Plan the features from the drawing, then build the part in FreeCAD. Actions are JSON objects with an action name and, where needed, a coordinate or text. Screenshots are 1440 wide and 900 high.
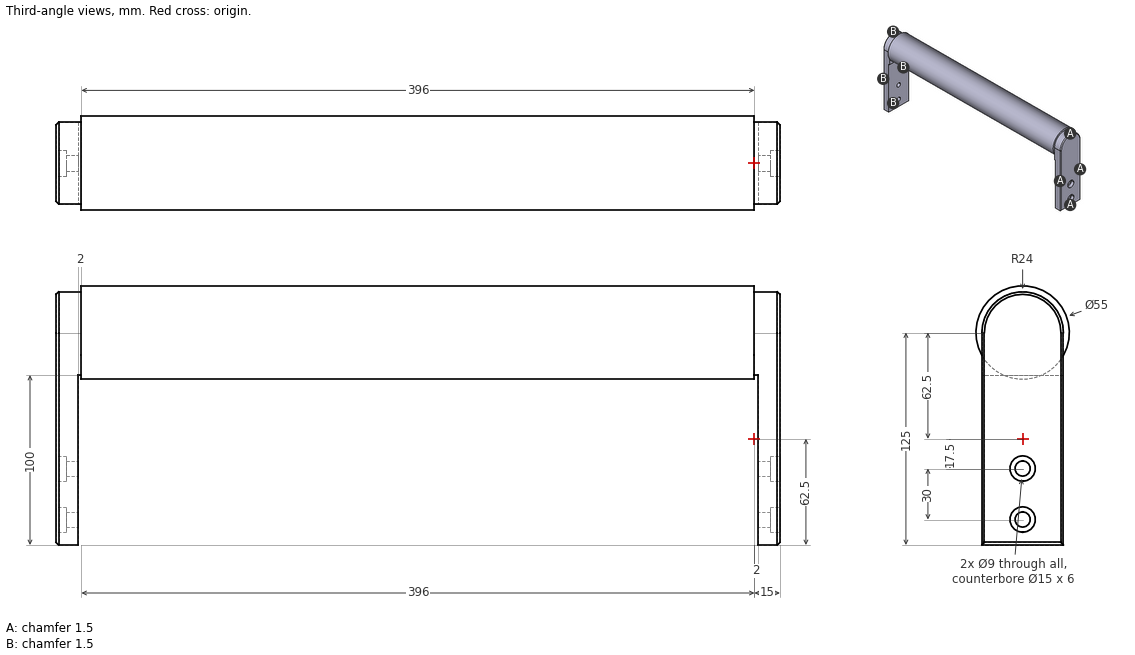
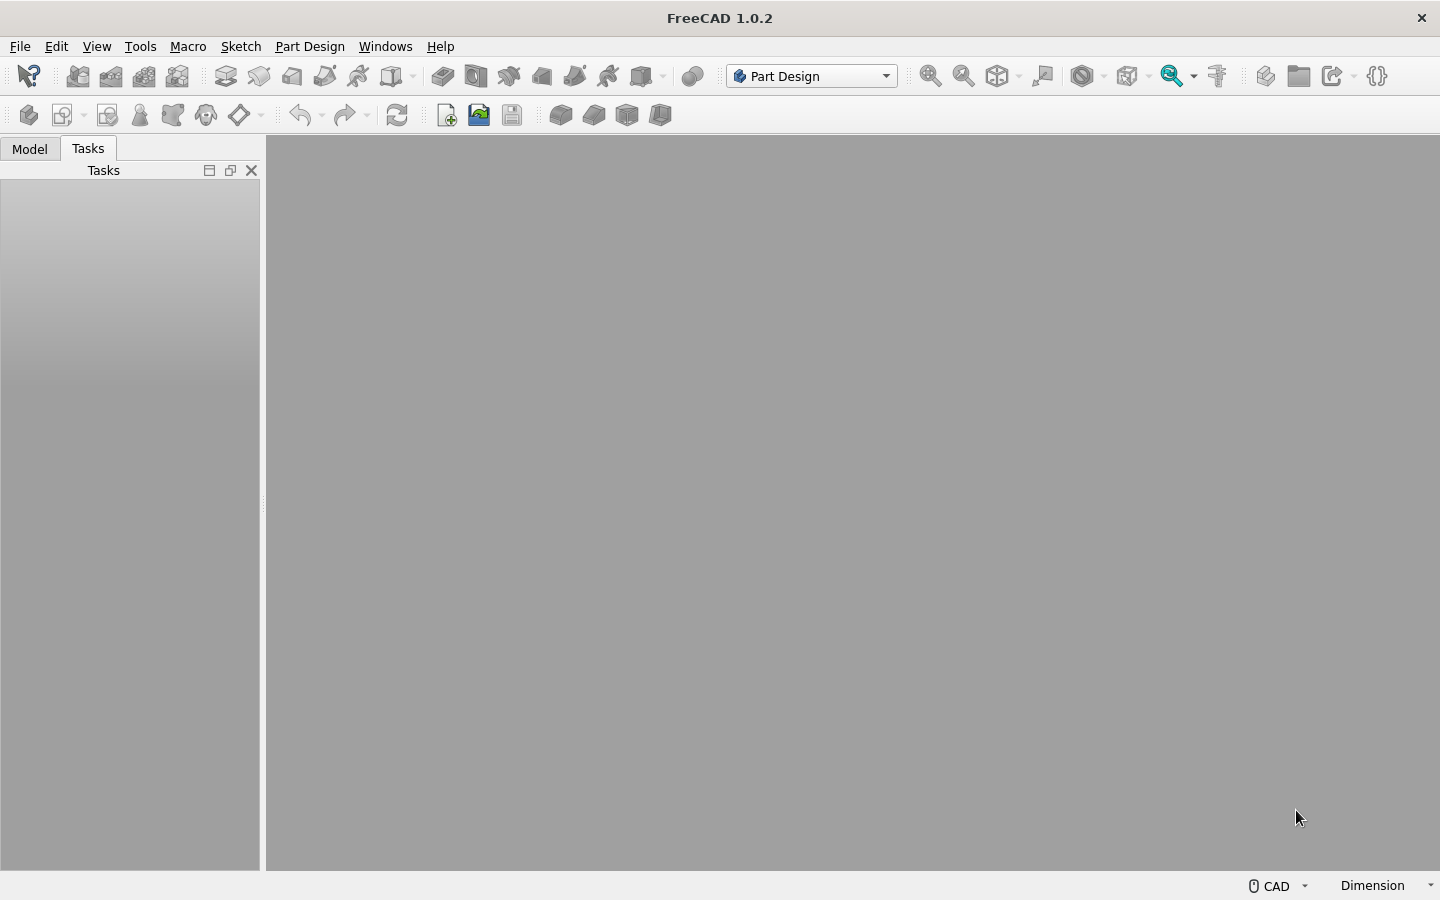
{"action": "left_click", "coordinate": [446, 116]}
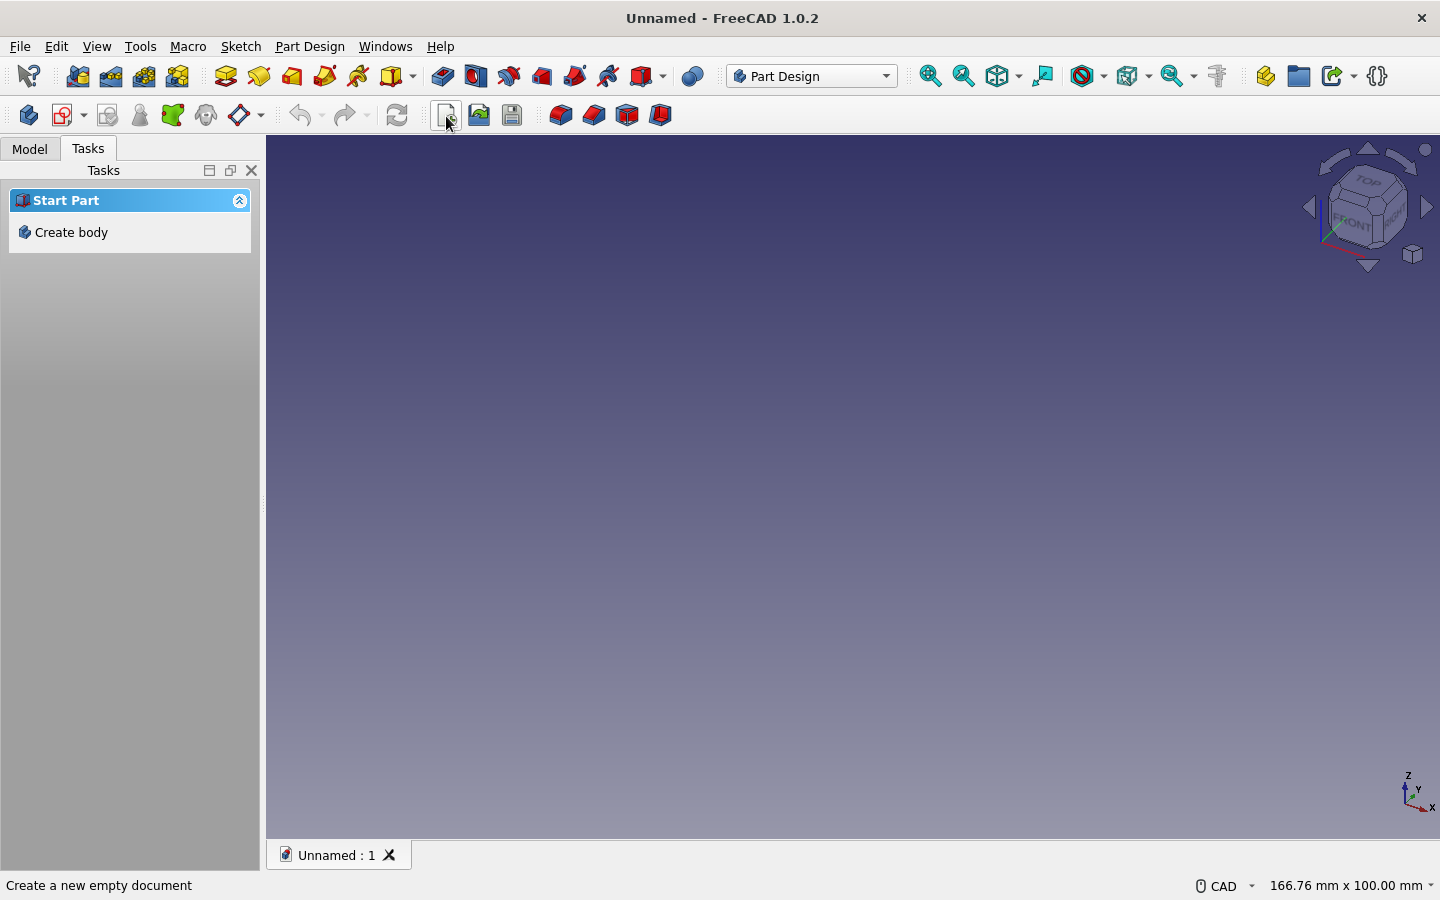
{"action": "left_click", "coordinate": [62, 116]}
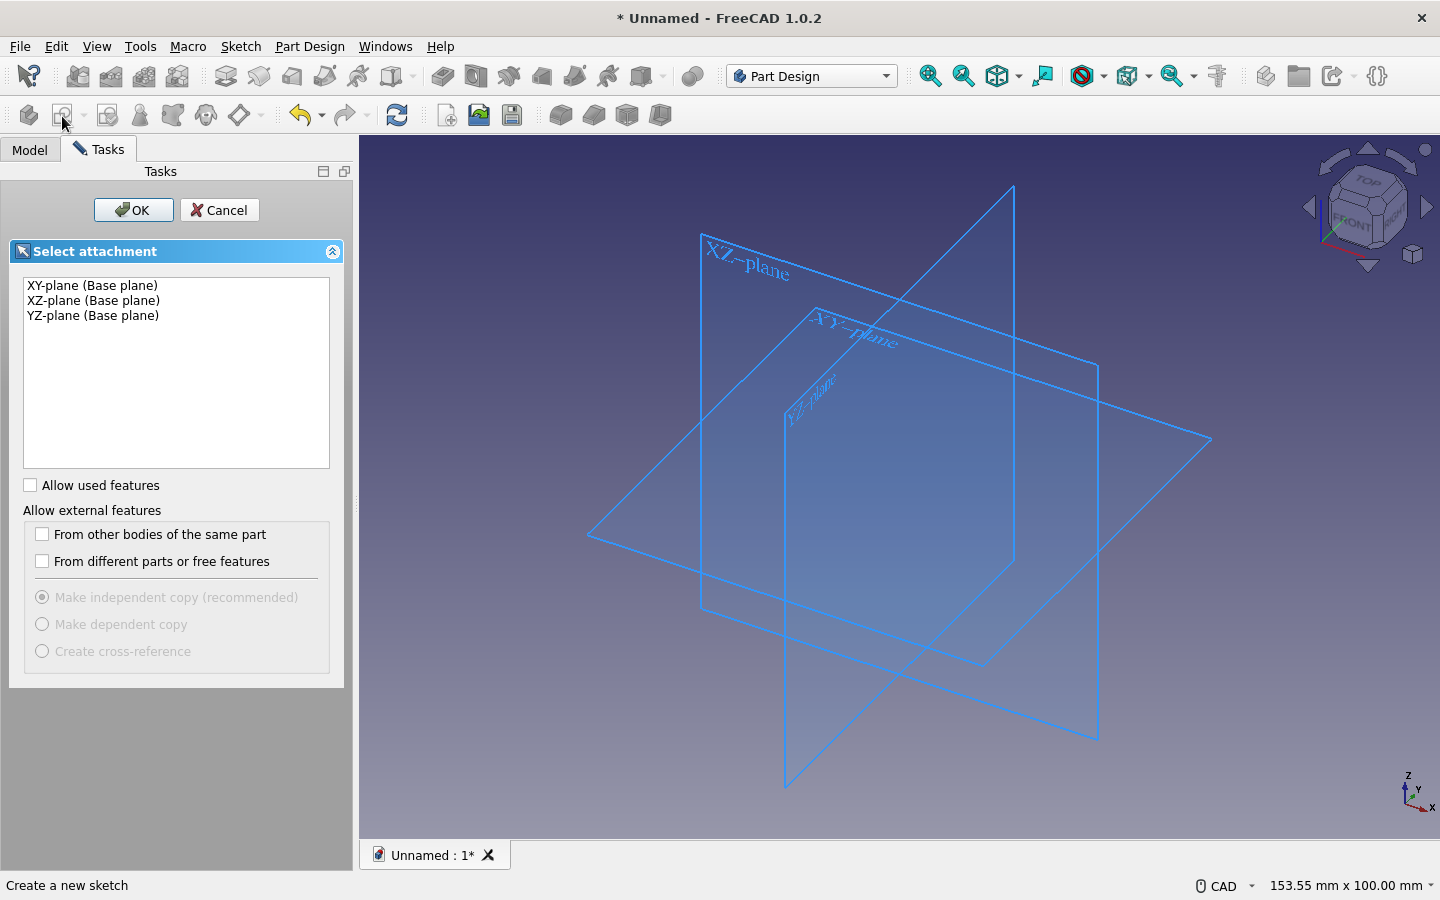
{"action": "left_click", "coordinate": [84, 316]}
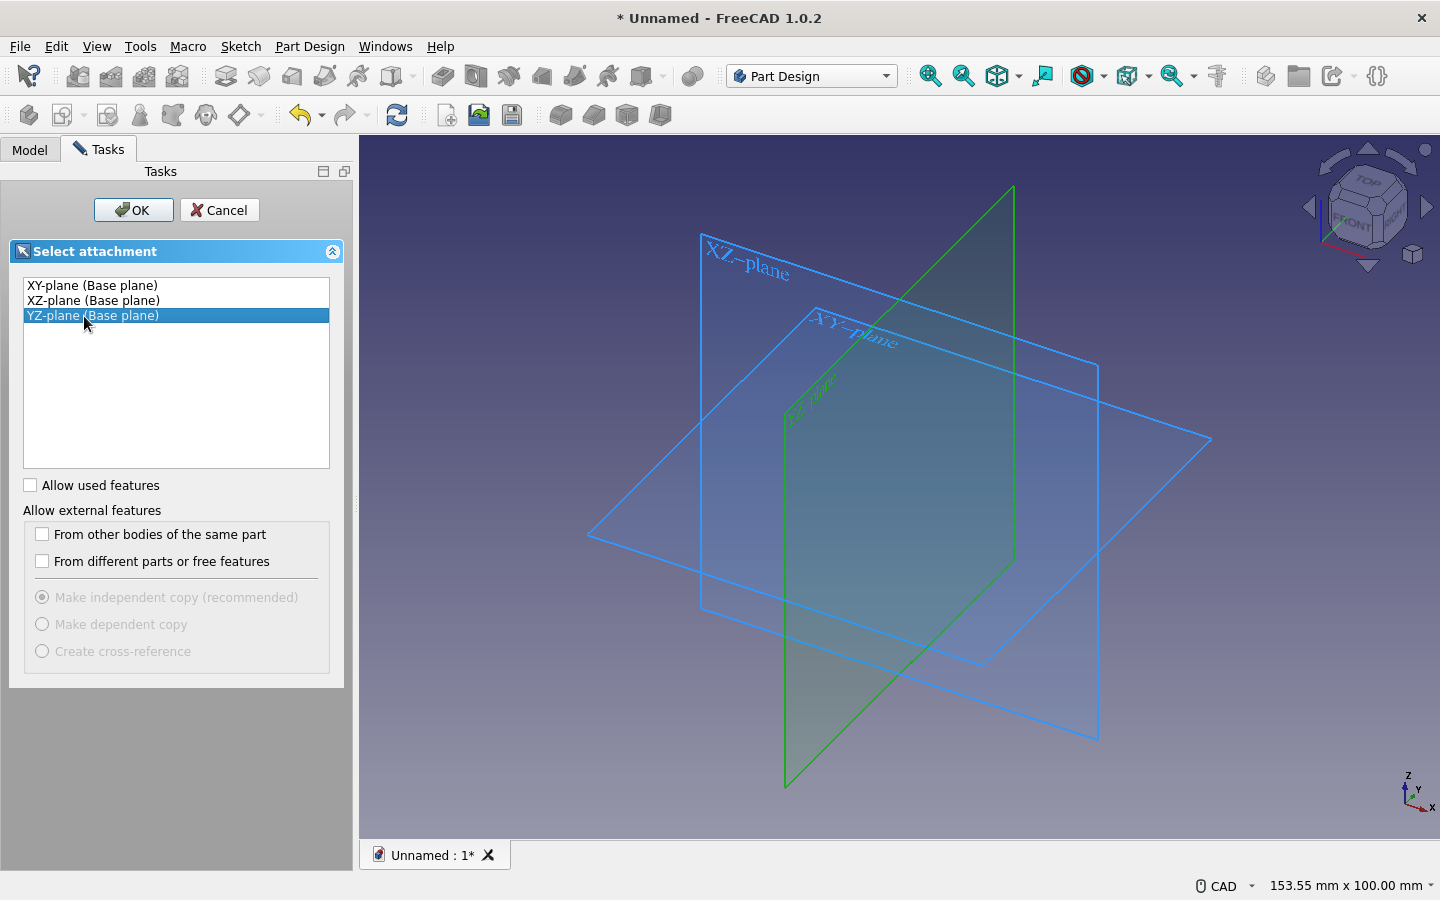
{"action": "left_click", "coordinate": [134, 210]}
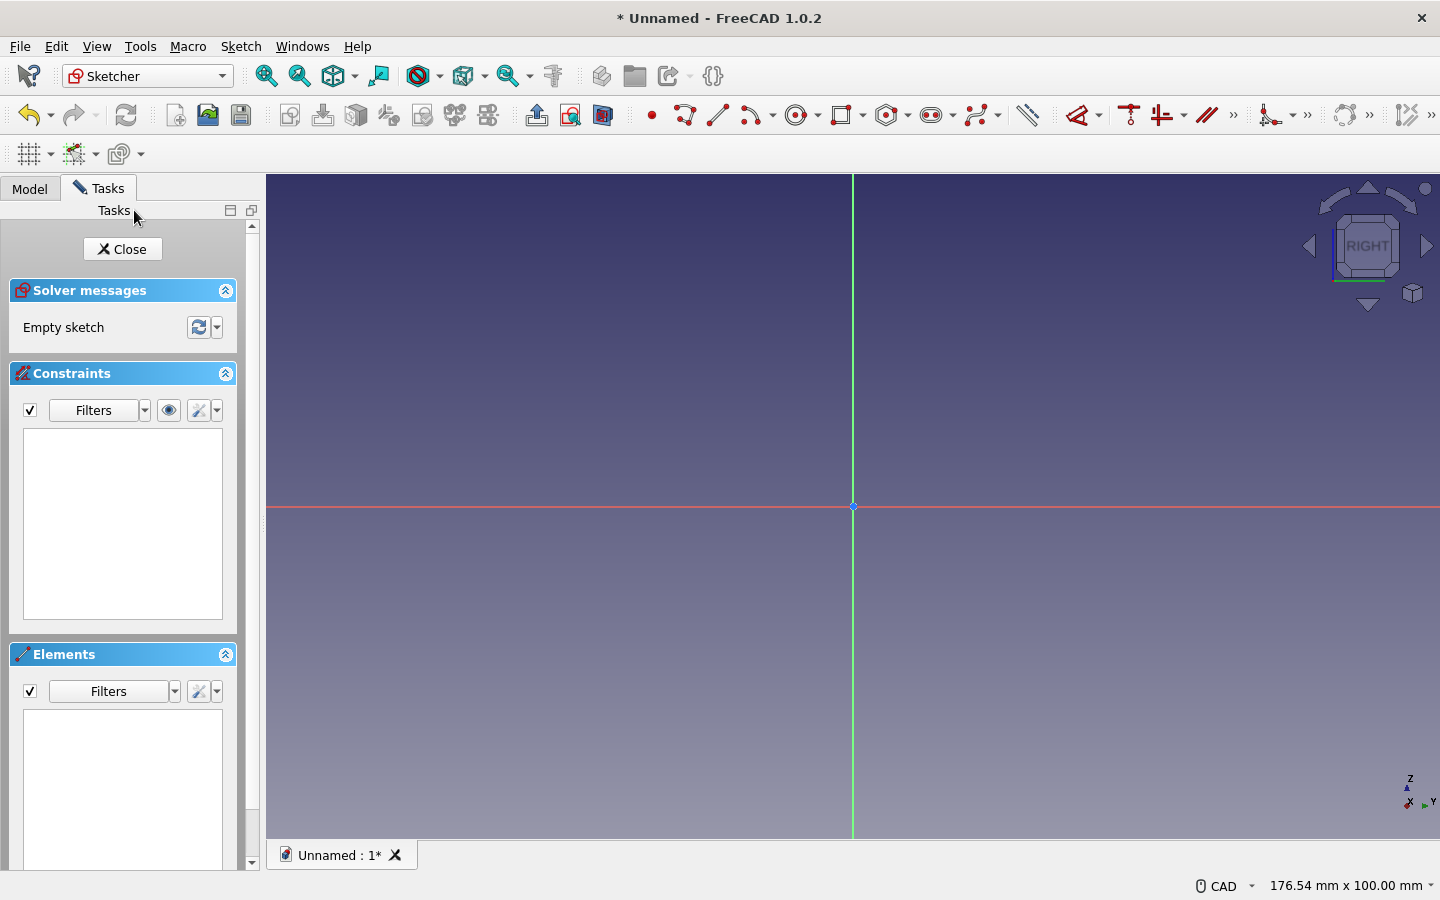
{"action": "scroll", "coordinate": [729, 572], "scroll_direction": "down", "scroll_amount": 4}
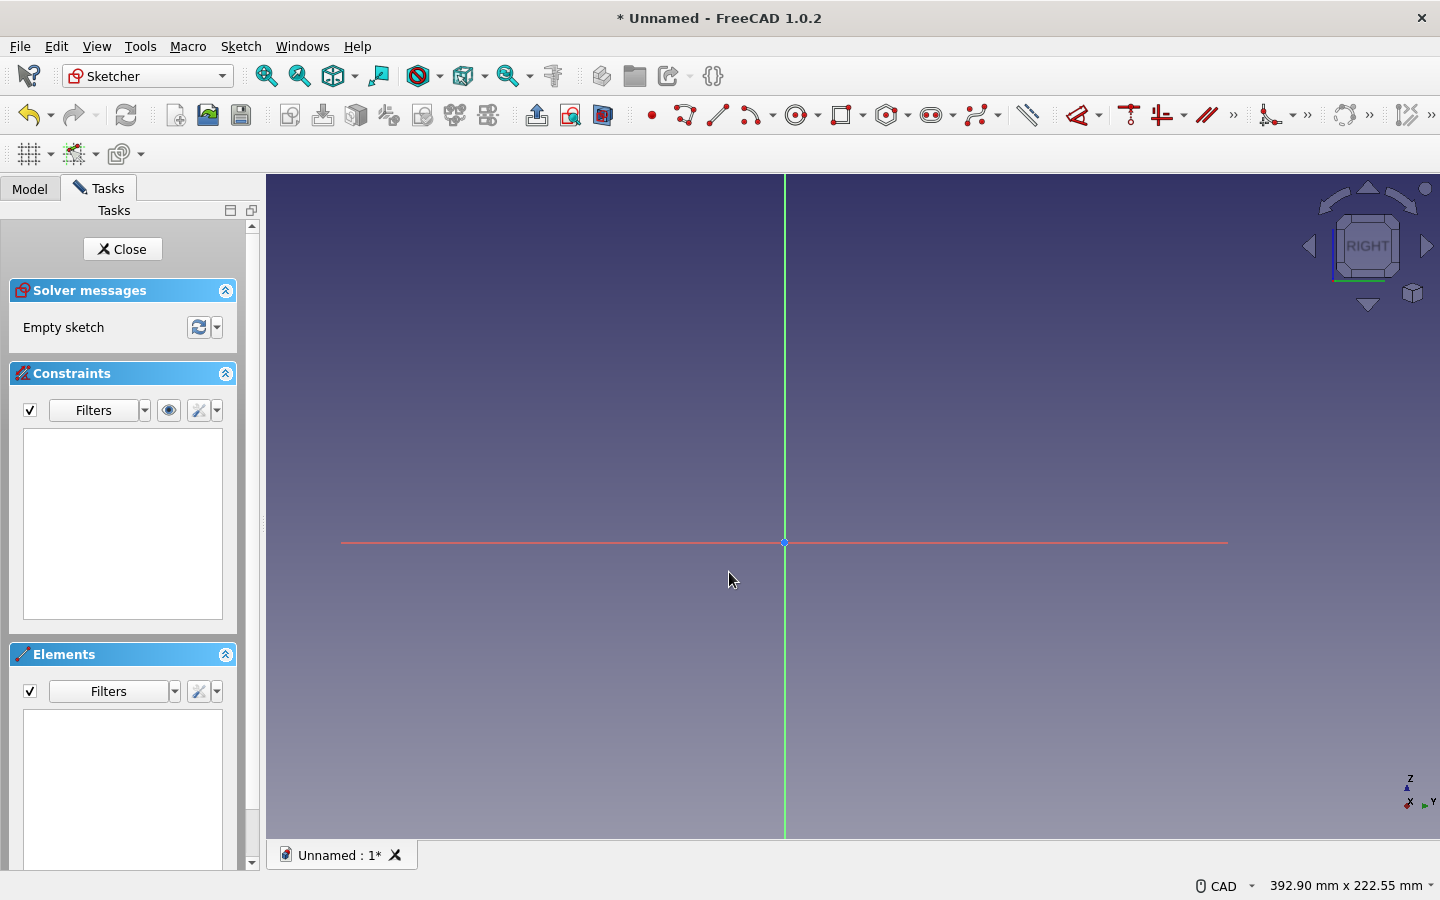
{"action": "left_click", "coordinate": [685, 116]}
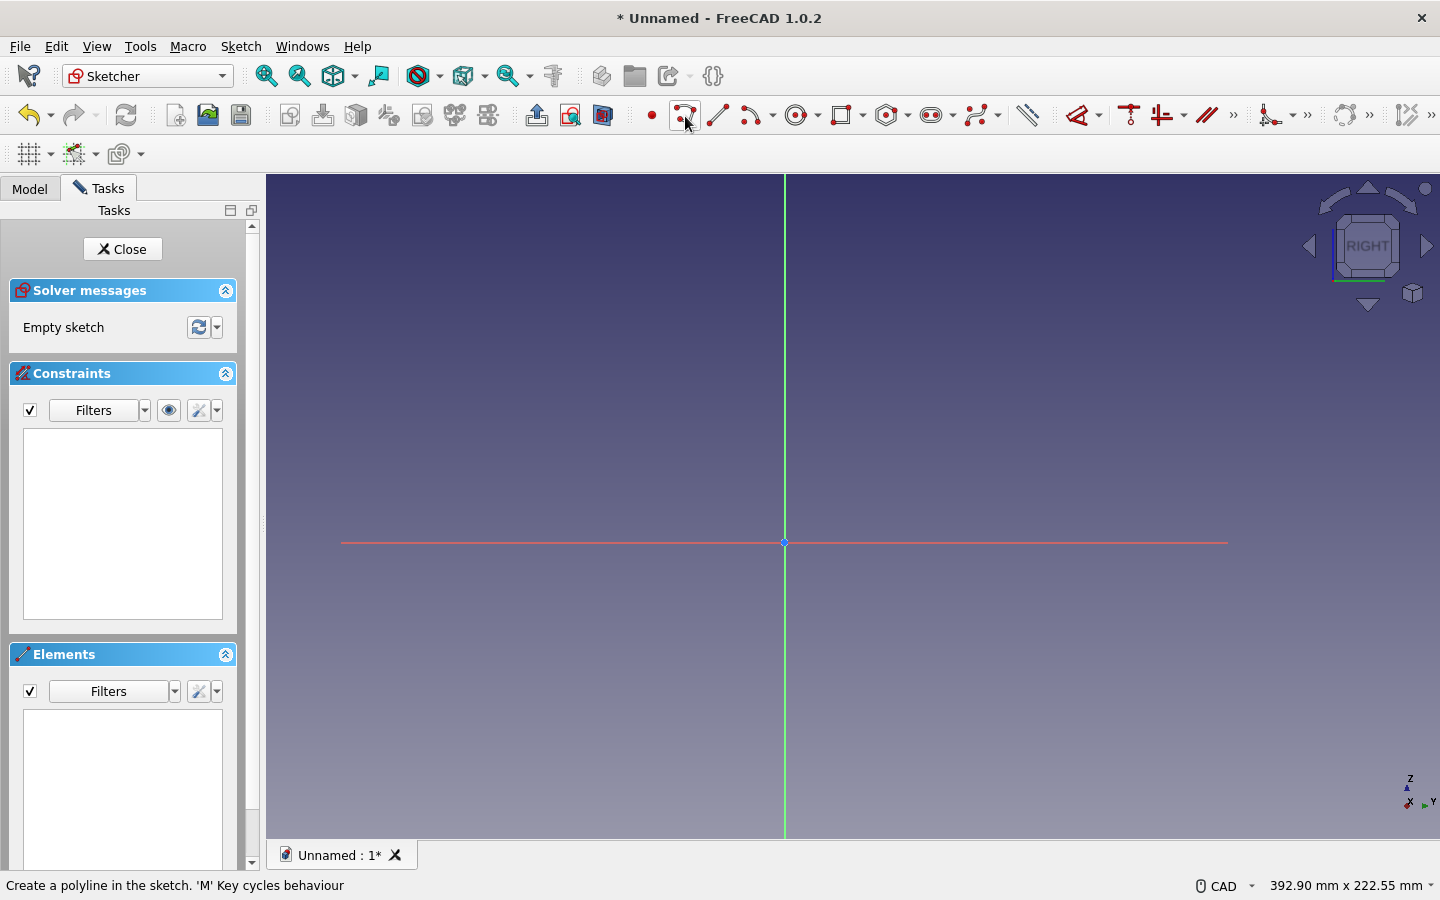
{"action": "left_click", "coordinate": [713, 356]}
{"action": "left_click", "coordinate": [713, 730]}
{"action": "left_click", "coordinate": [857, 730]}
{"action": "left_click", "coordinate": [857, 356]}
{"action": "right_click", "coordinate": [857, 356]}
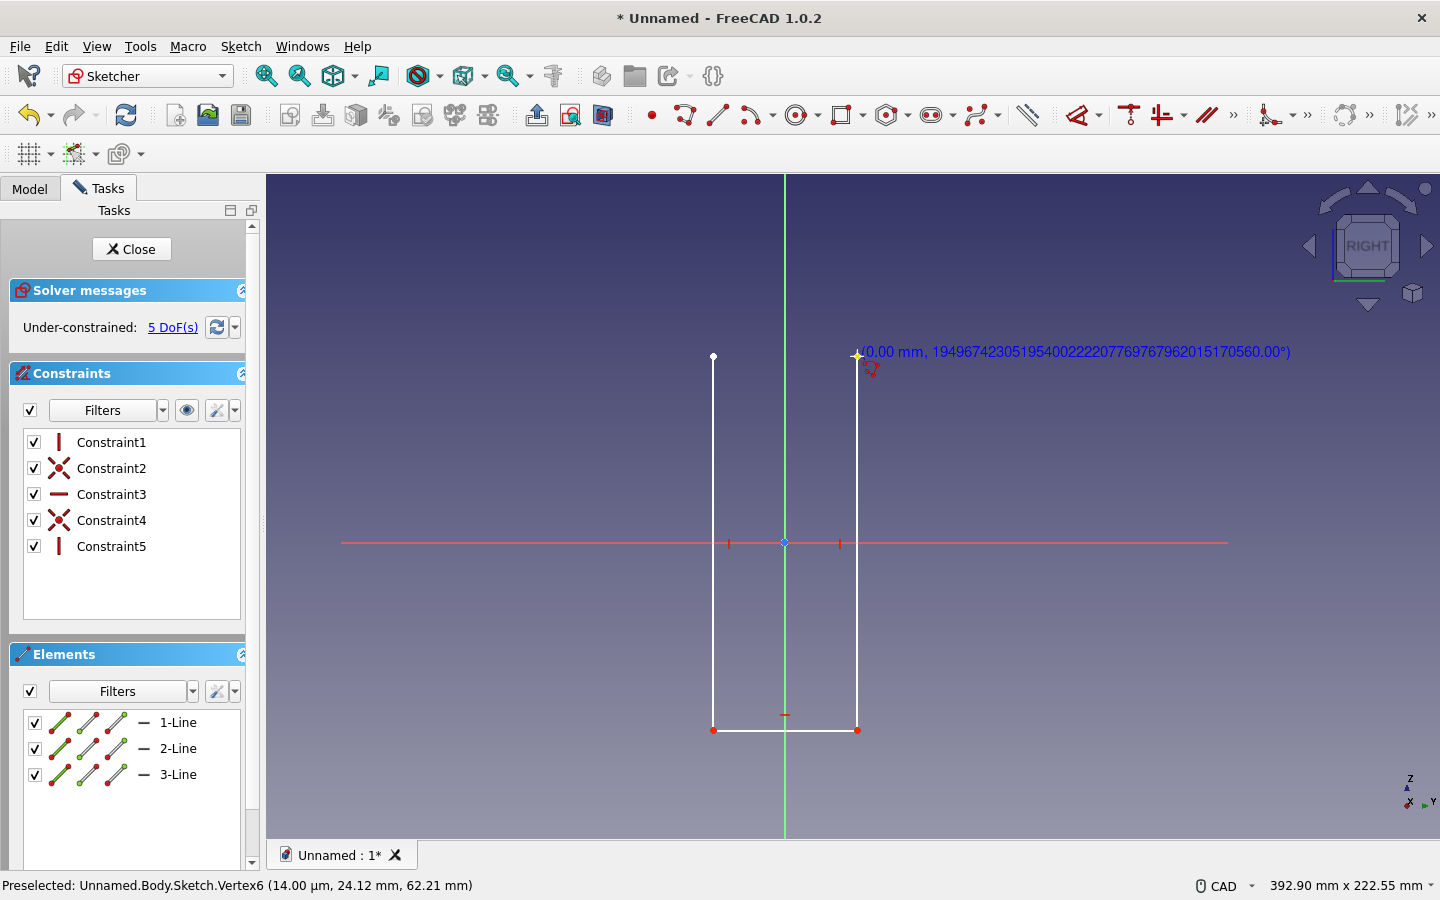
{"action": "key", "text": "g 3 a"}